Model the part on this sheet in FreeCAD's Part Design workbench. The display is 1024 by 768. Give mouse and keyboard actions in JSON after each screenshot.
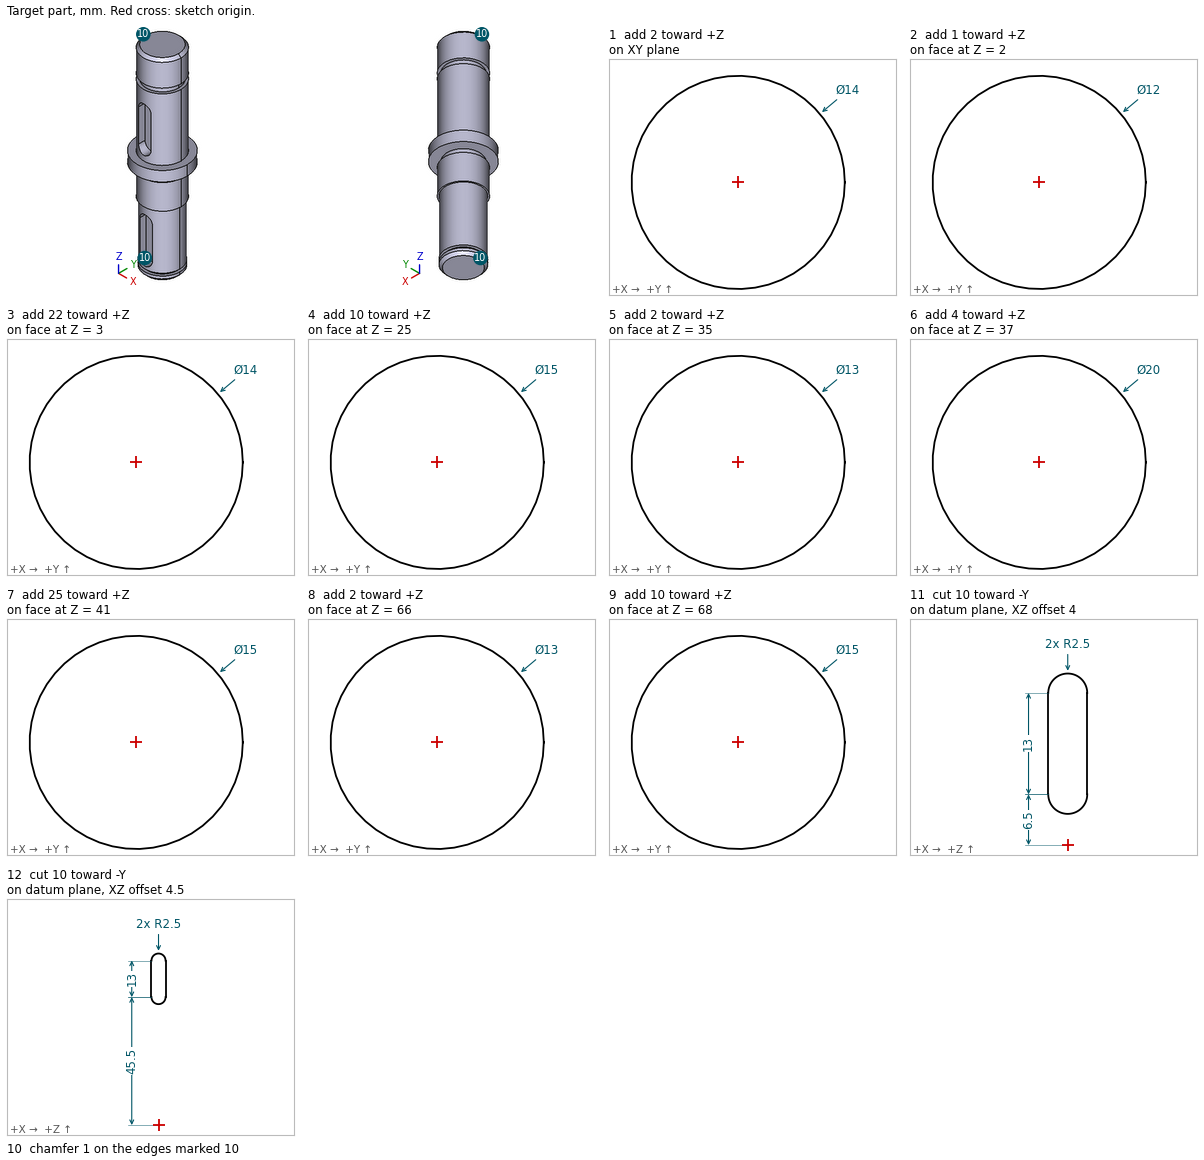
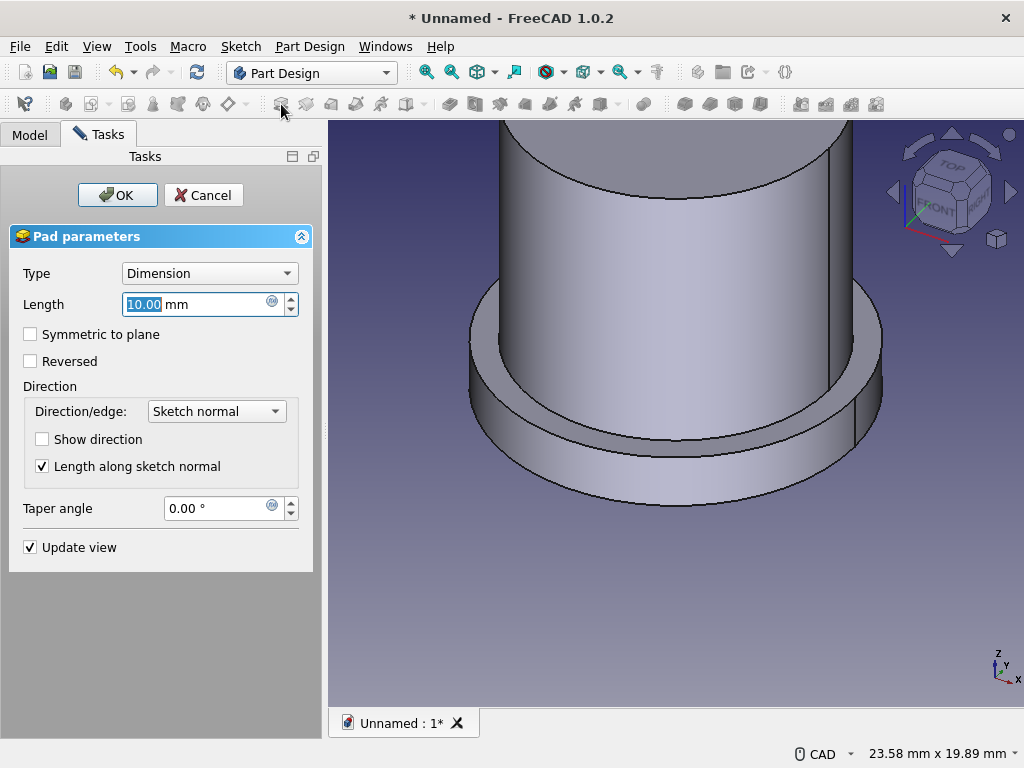
{"action": "type", "text": "1"}
{"action": "key", "text": "Tab"}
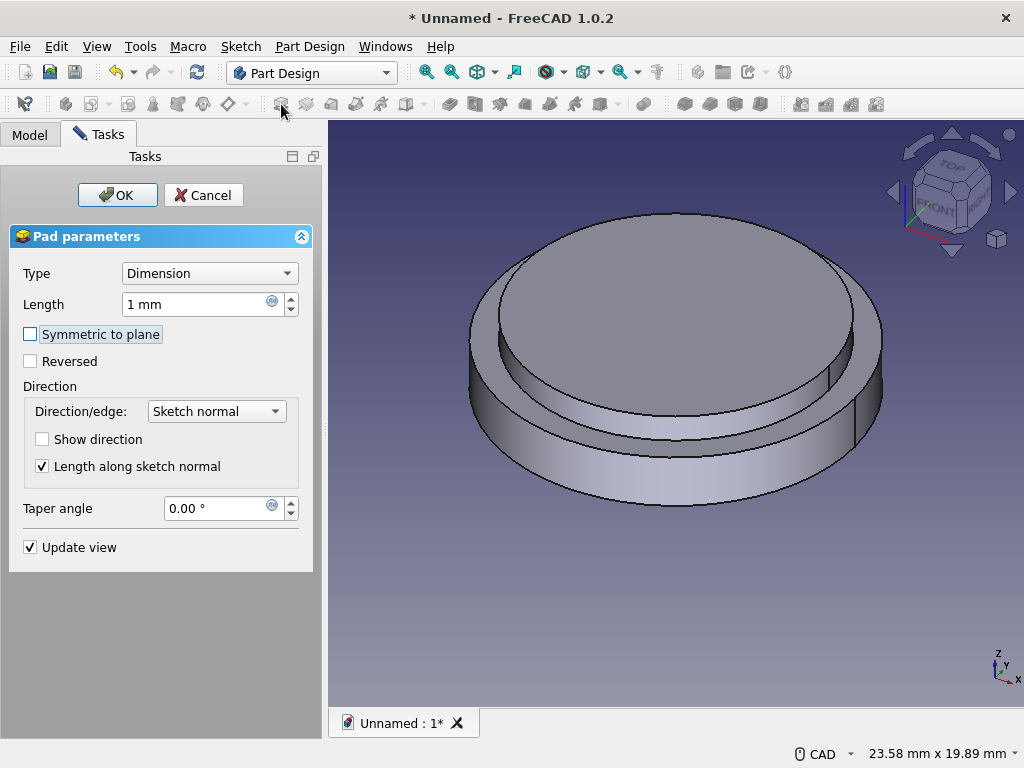
{"action": "left_click", "coordinate": [118, 195]}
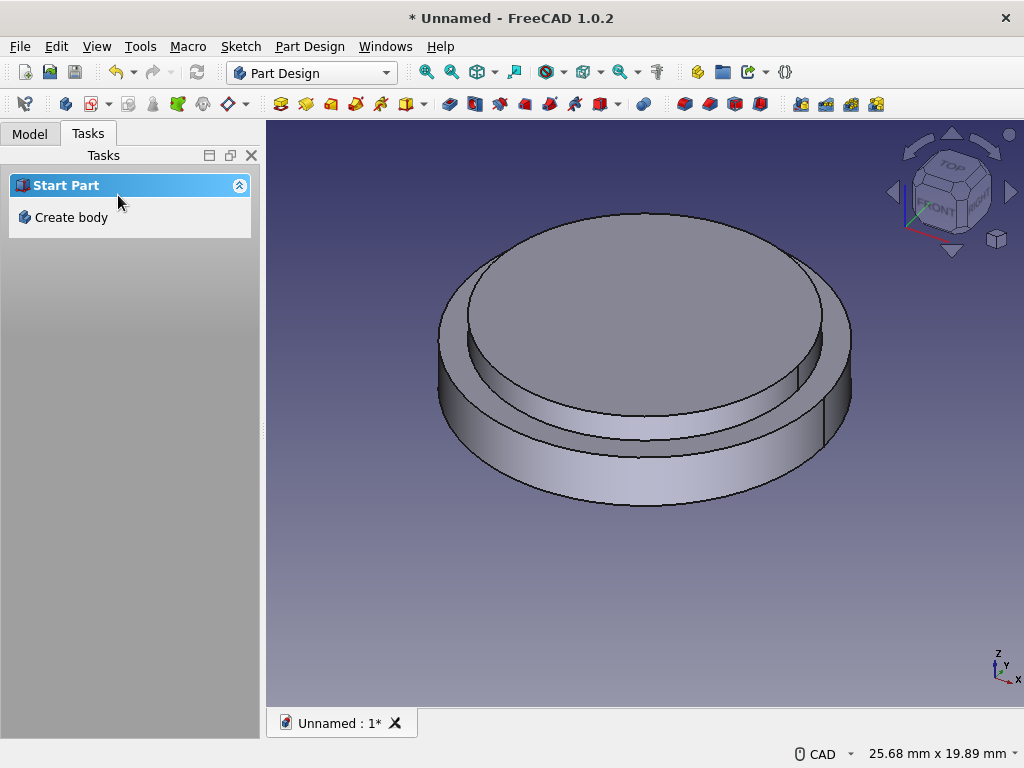
{"action": "left_click", "coordinate": [645, 314]}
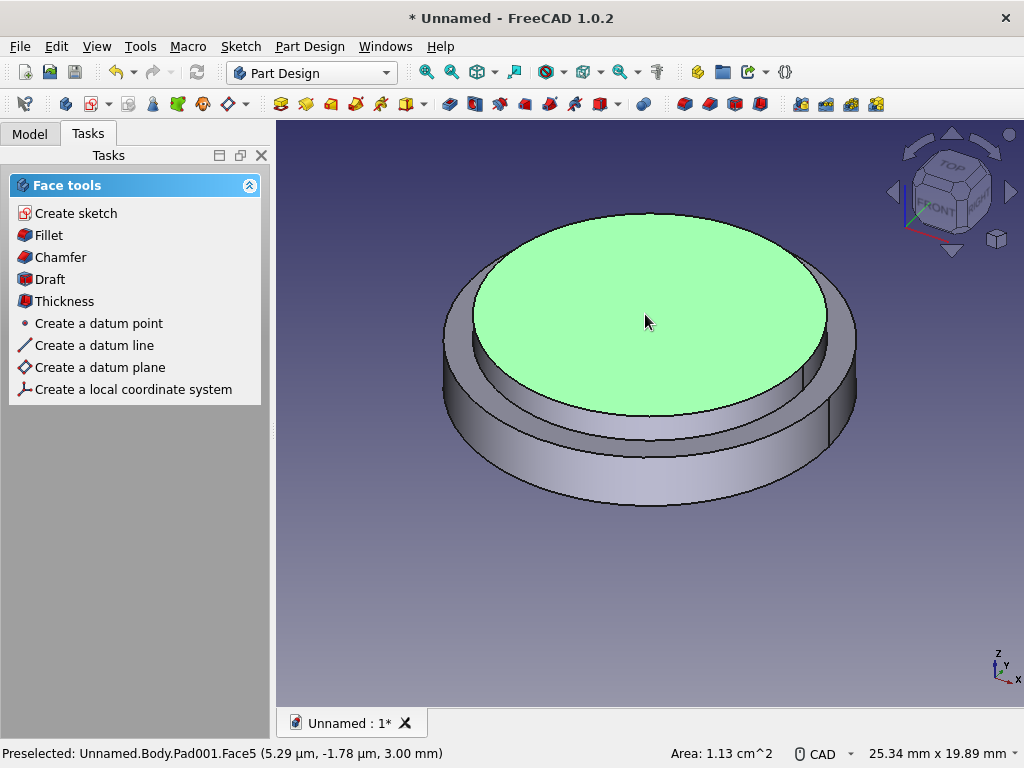
{"action": "left_click", "coordinate": [90, 104]}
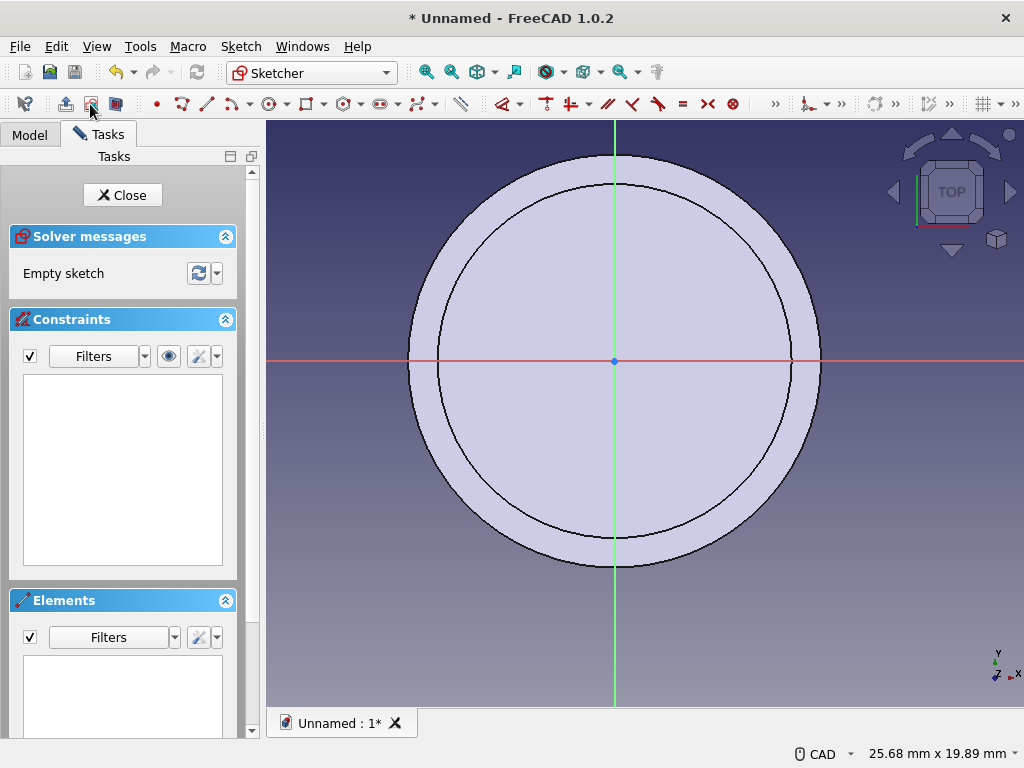
{"action": "scroll", "coordinate": [404, 650], "scroll_direction": "down", "scroll_amount": 1}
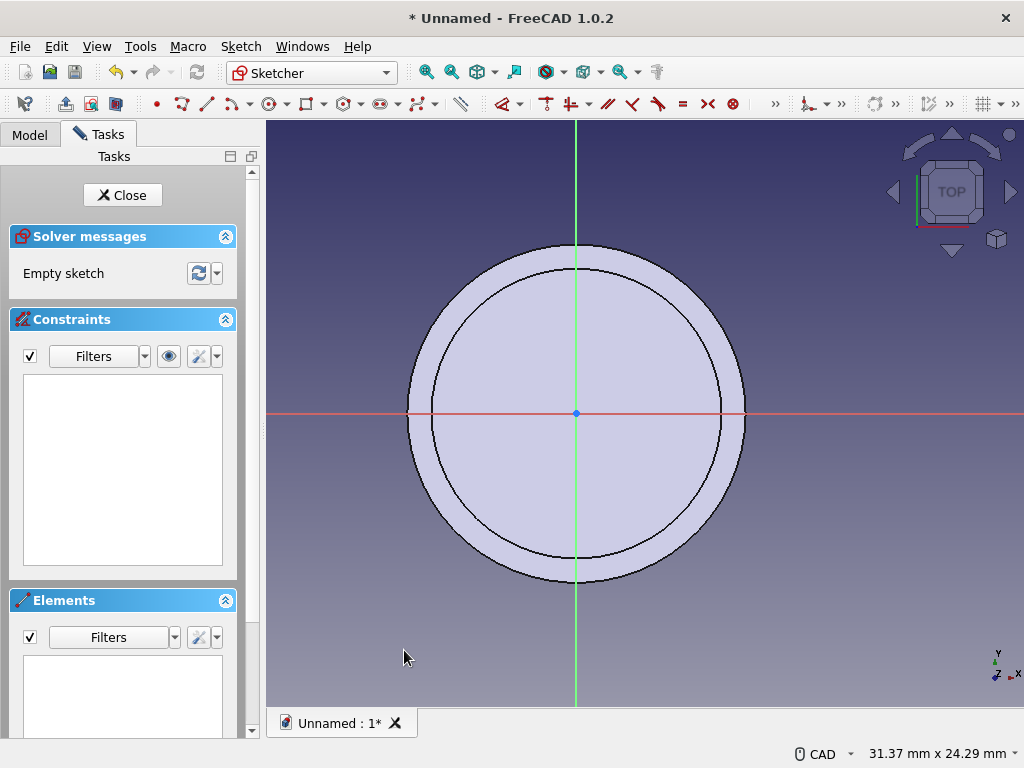
{"action": "left_click", "coordinate": [268, 104]}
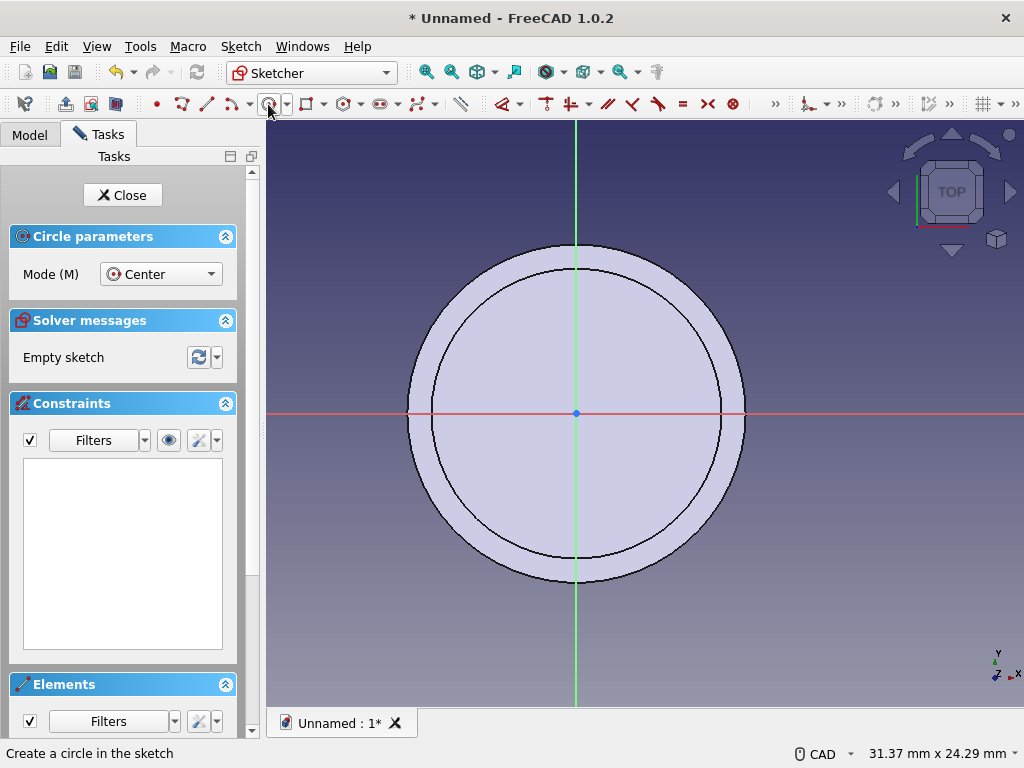
{"action": "left_click", "coordinate": [576, 414]}
{"action": "left_click", "coordinate": [696, 294]}
{"action": "key", "text": "Escape"}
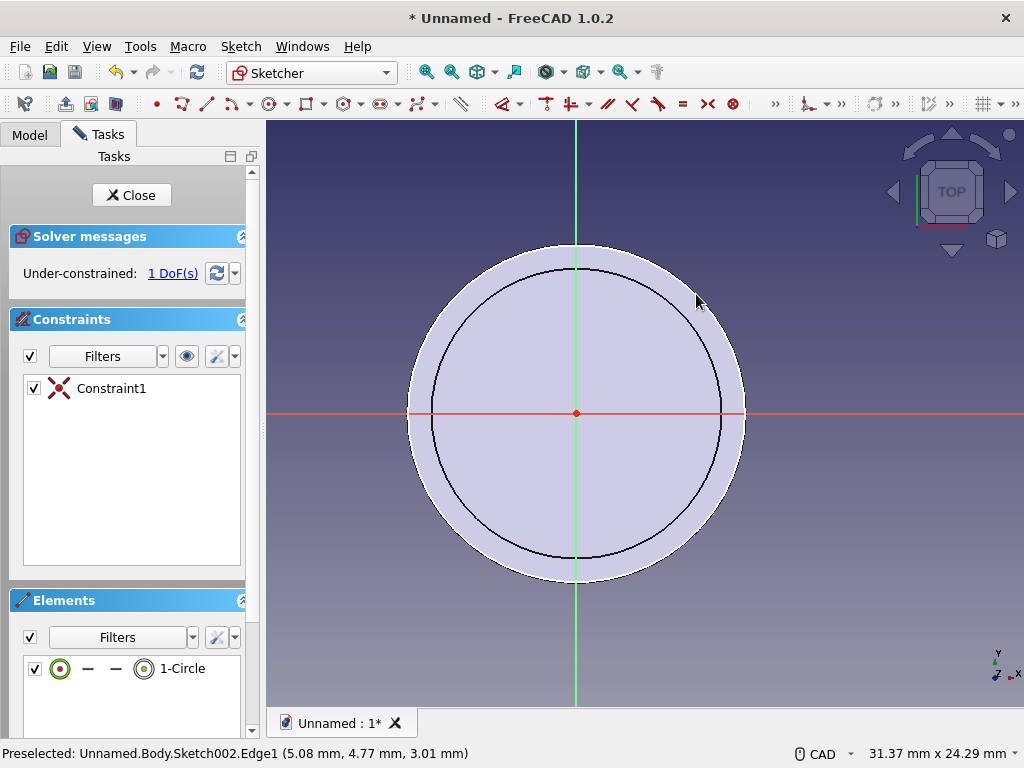
{"action": "left_click", "coordinate": [502, 104]}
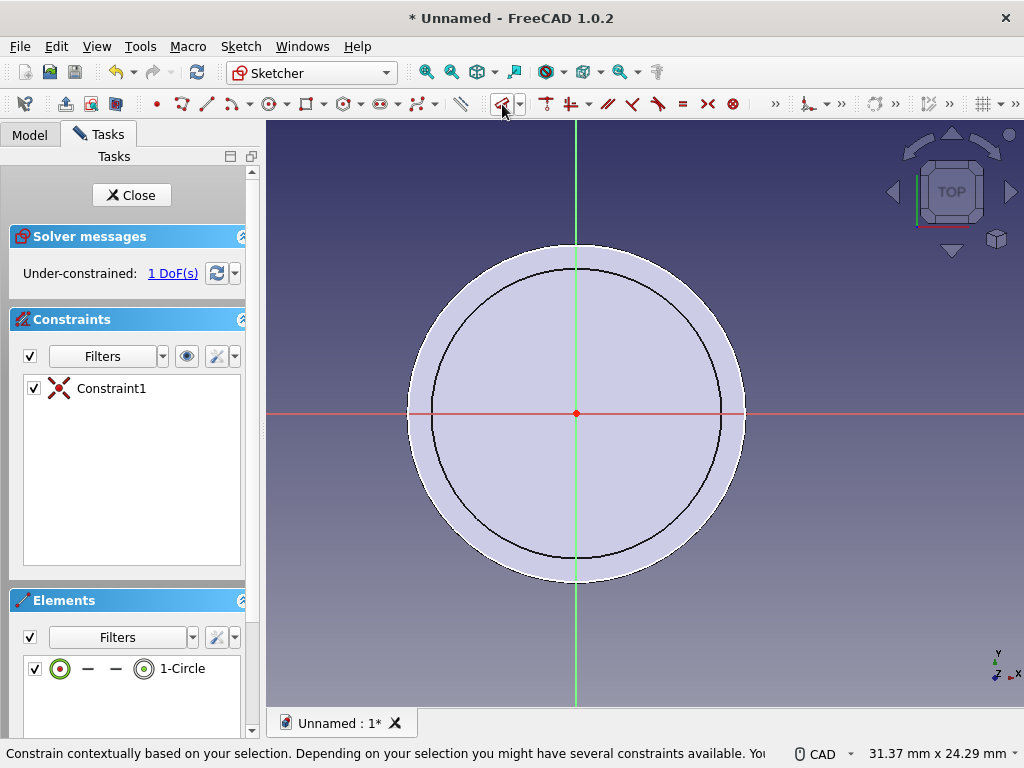
{"action": "left_click", "coordinate": [695, 294]}
{"action": "left_click", "coordinate": [718, 271]}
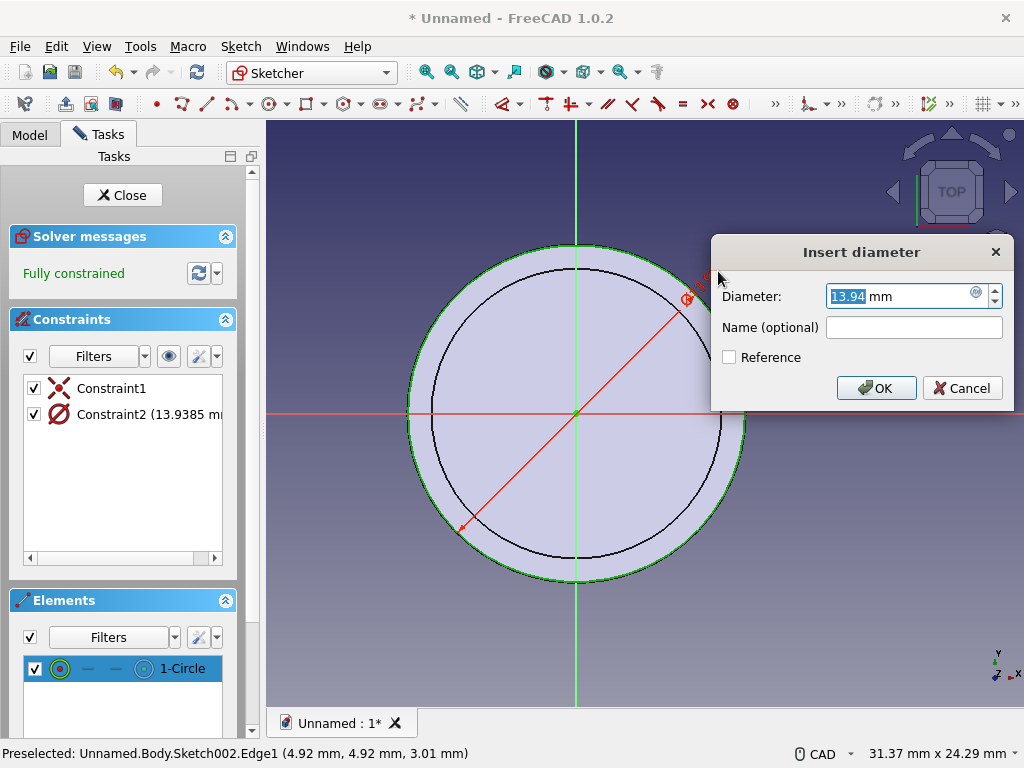
{"action": "type", "text": "14"}
{"action": "key", "text": "Return"}
{"action": "key", "text": "Escape"}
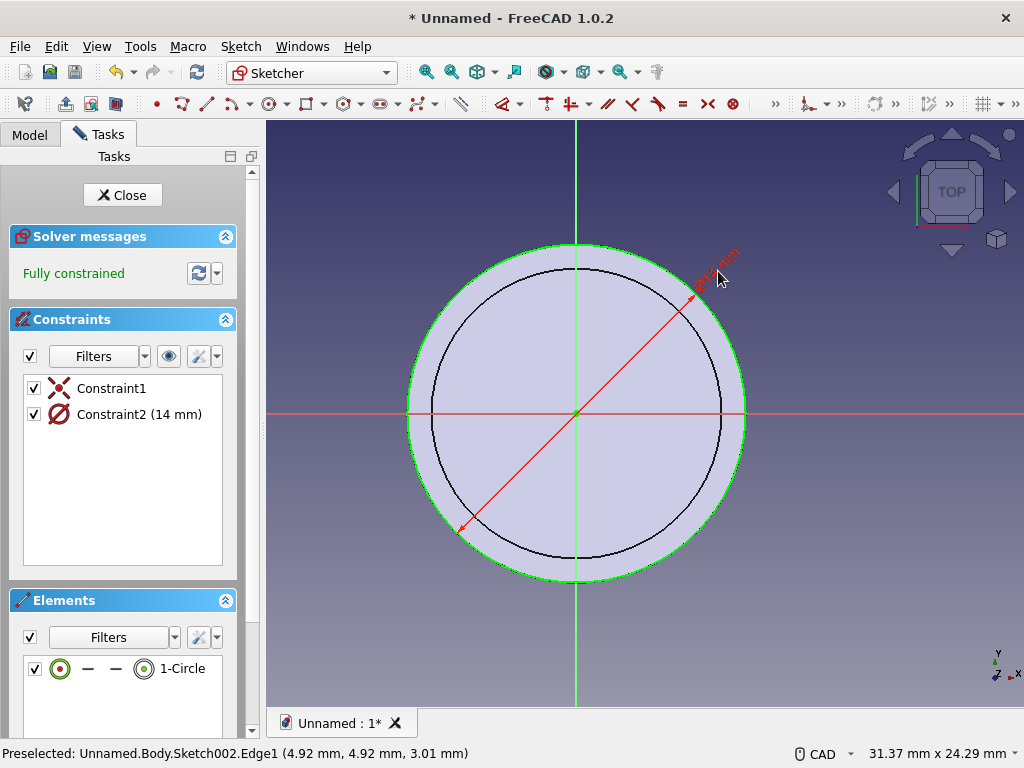
{"action": "left_click", "coordinate": [123, 195]}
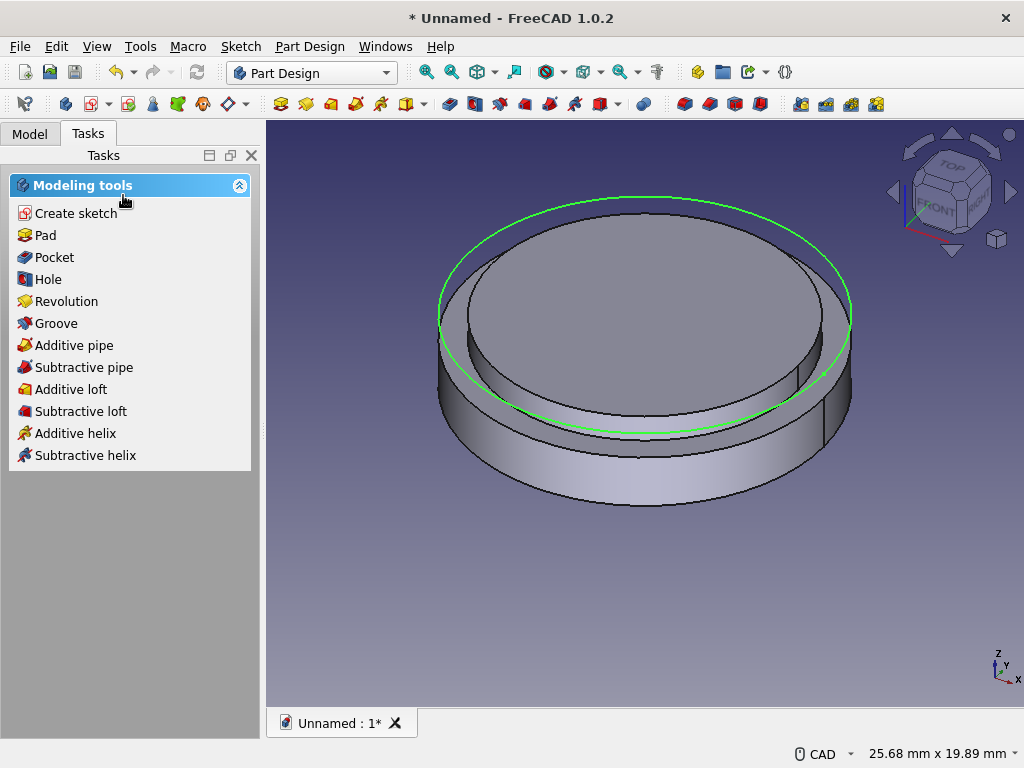
{"action": "left_click", "coordinate": [281, 104]}